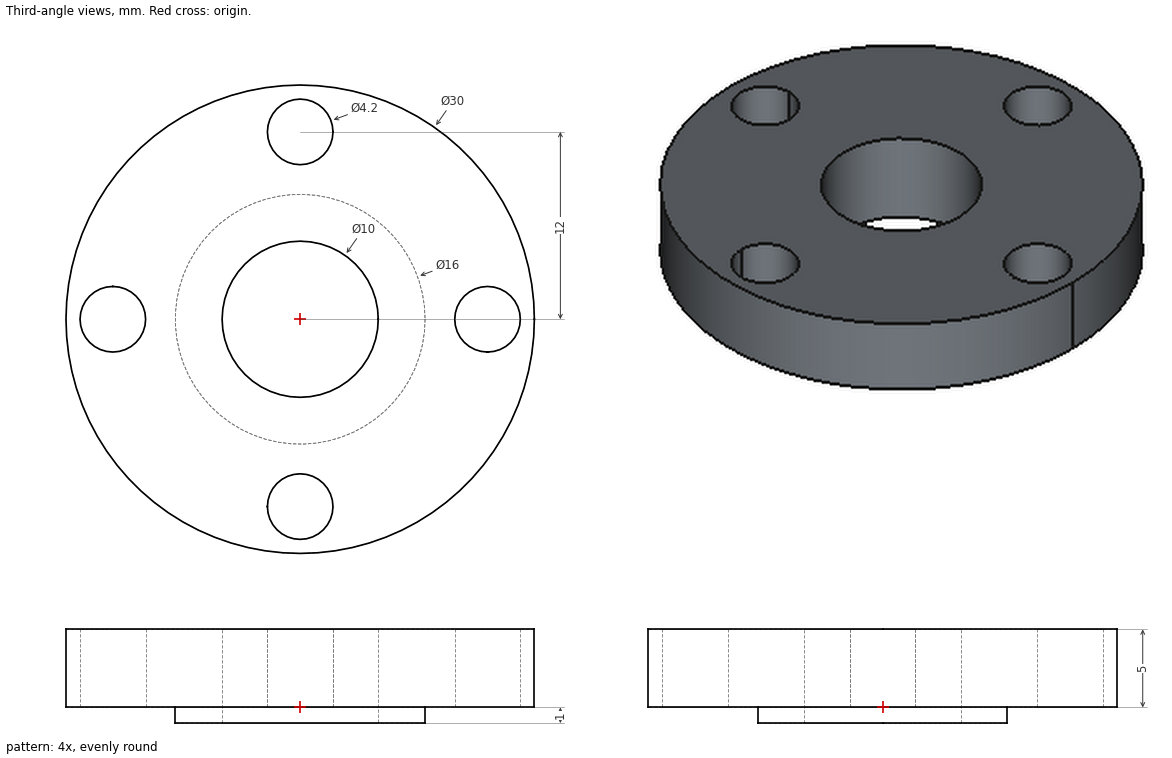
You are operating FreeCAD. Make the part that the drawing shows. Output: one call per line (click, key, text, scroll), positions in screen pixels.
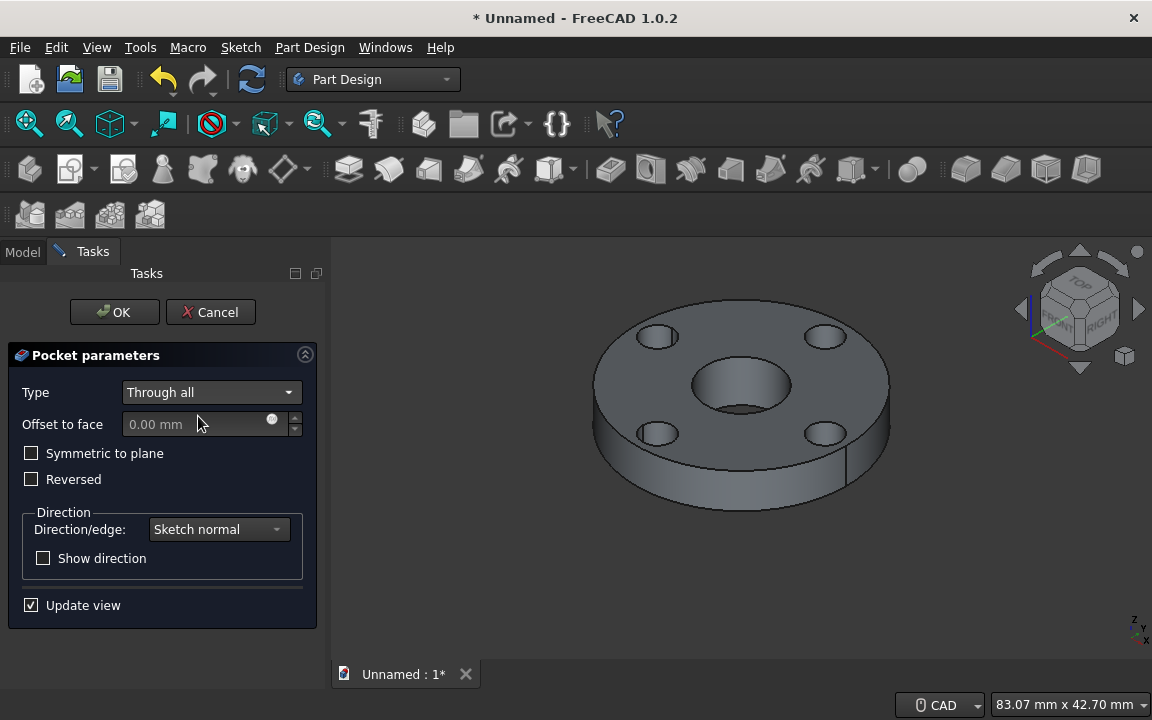
click(115, 312)